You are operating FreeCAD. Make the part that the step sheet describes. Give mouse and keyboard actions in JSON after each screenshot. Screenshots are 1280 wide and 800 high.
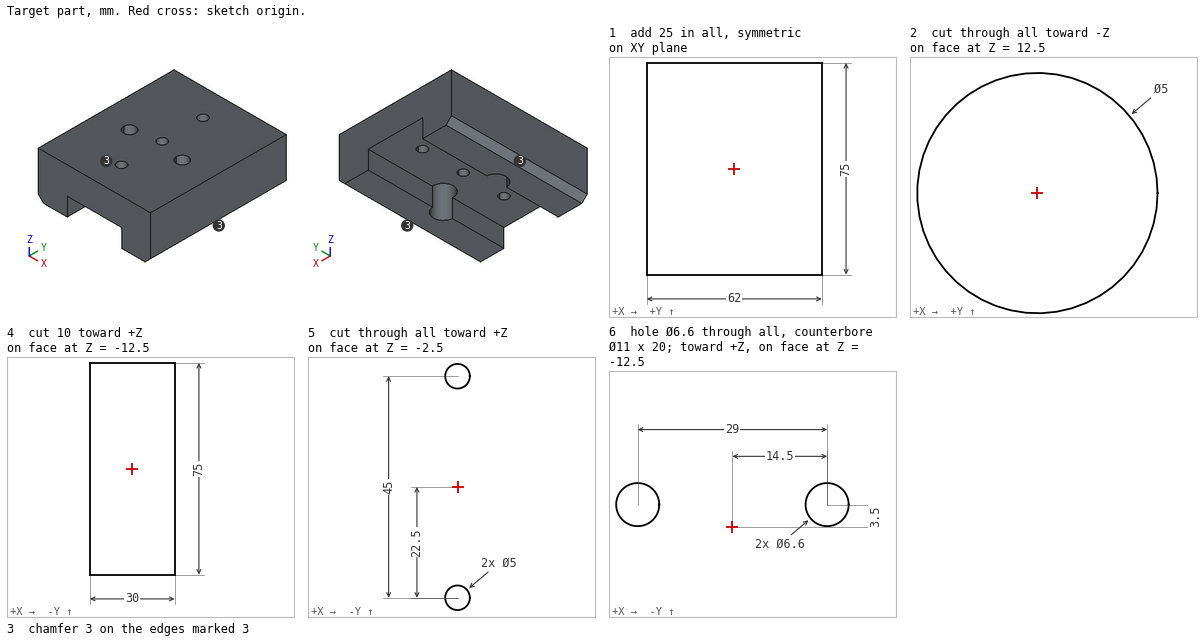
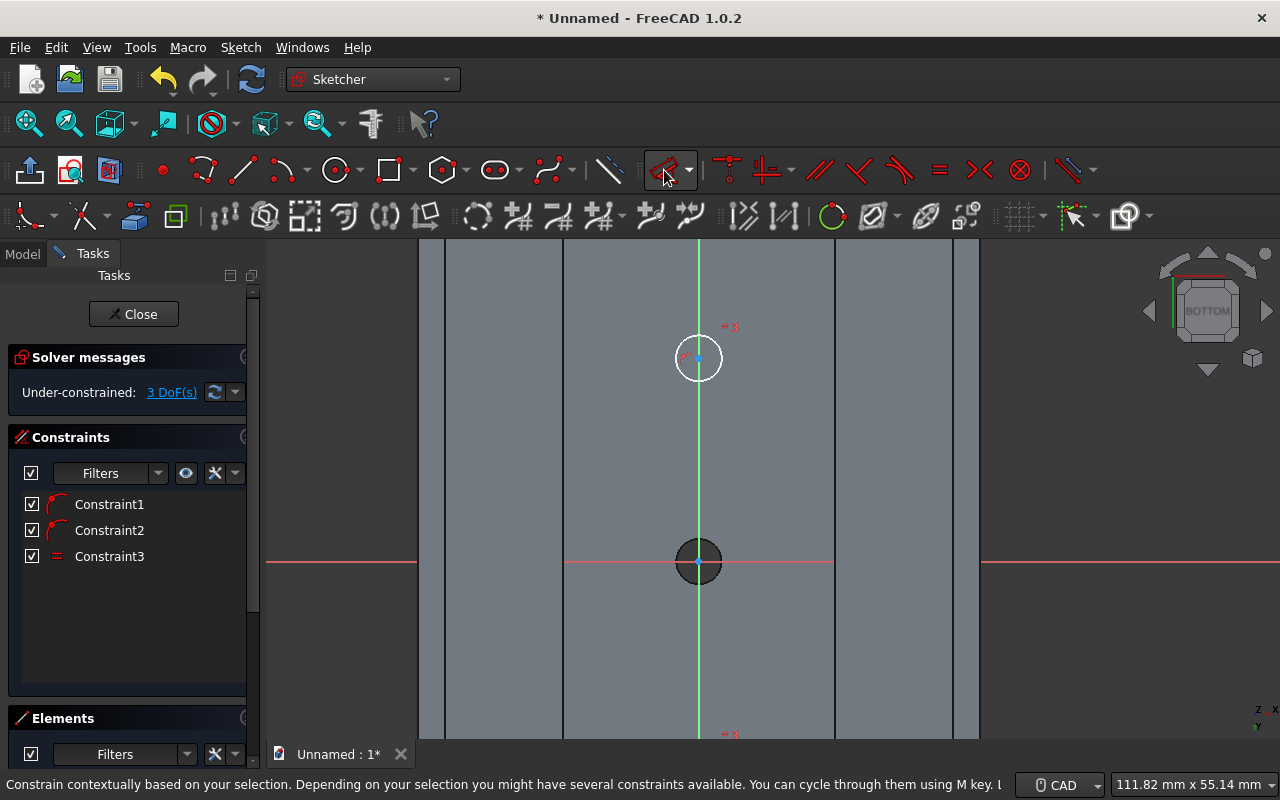
{"action": "scroll", "coordinate": [716, 341], "scroll_direction": "down", "scroll_amount": 2}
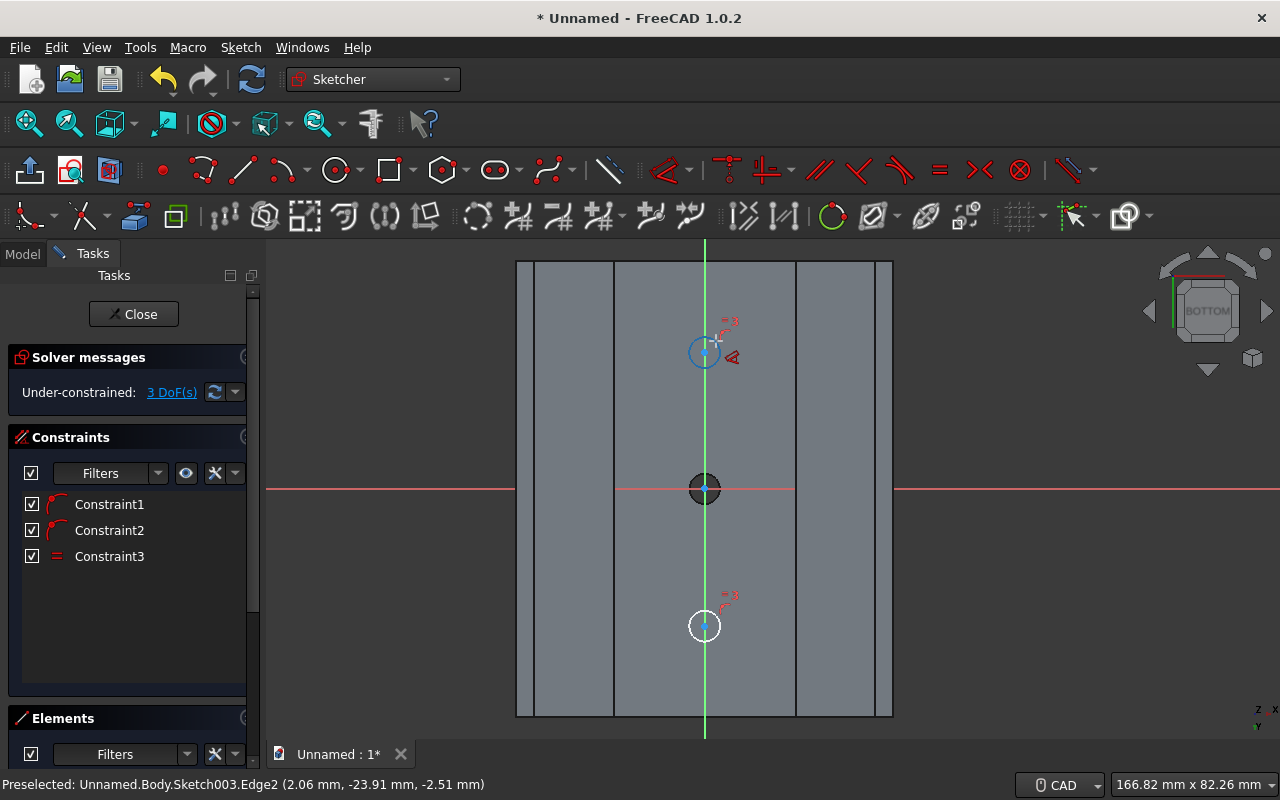
{"action": "scroll", "coordinate": [716, 615], "scroll_direction": "up", "scroll_amount": 2}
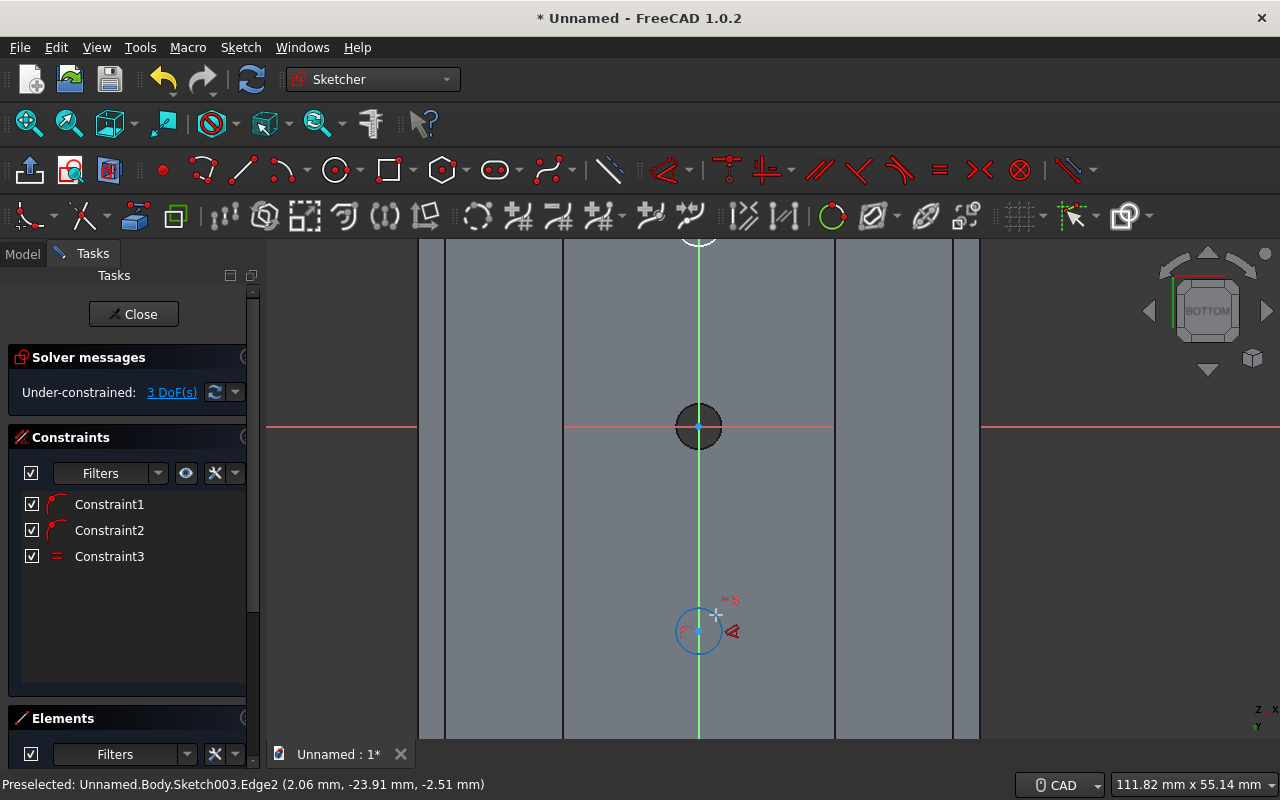
{"action": "left_click", "coordinate": [715, 615]}
{"action": "left_click", "coordinate": [737, 592]}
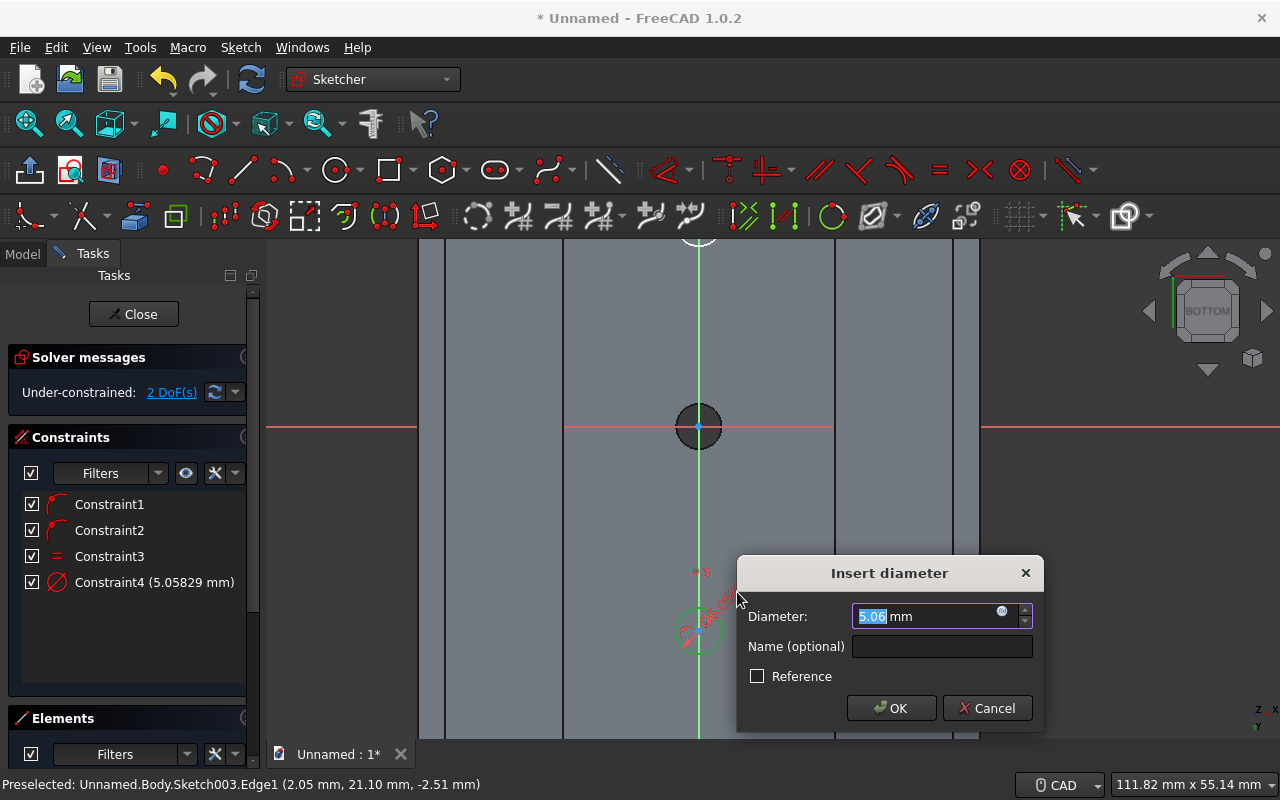
{"action": "type", "text": "5"}
{"action": "key", "text": "Return"}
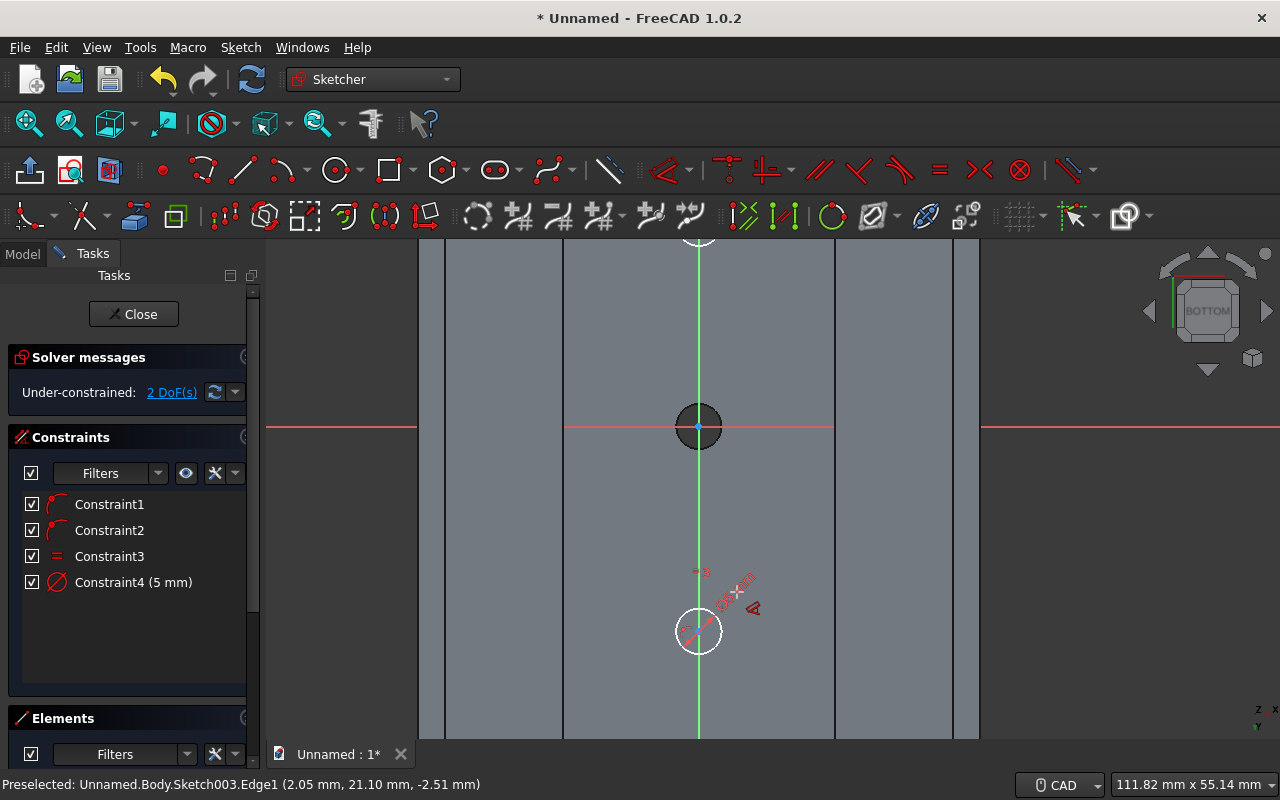
{"action": "left_click", "coordinate": [699, 631]}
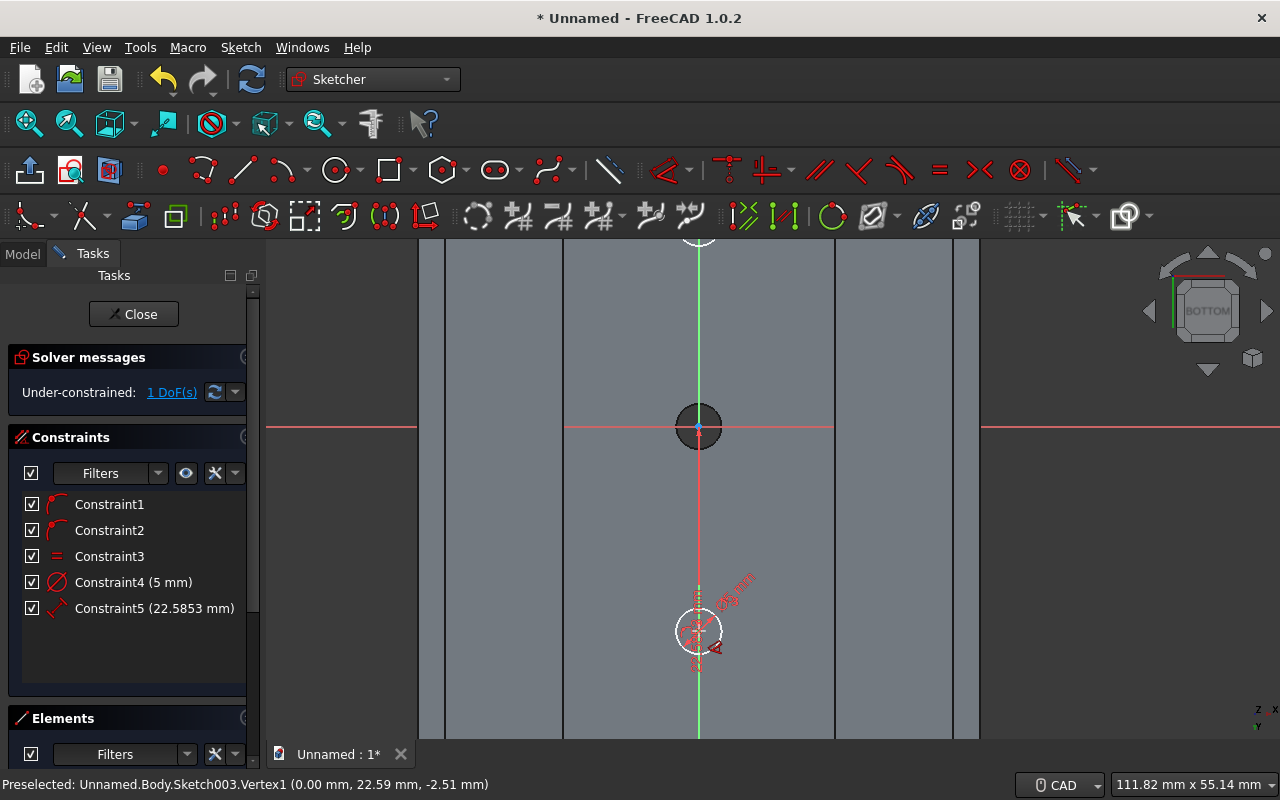
{"action": "scroll", "coordinate": [716, 616], "scroll_direction": "down", "scroll_amount": 2}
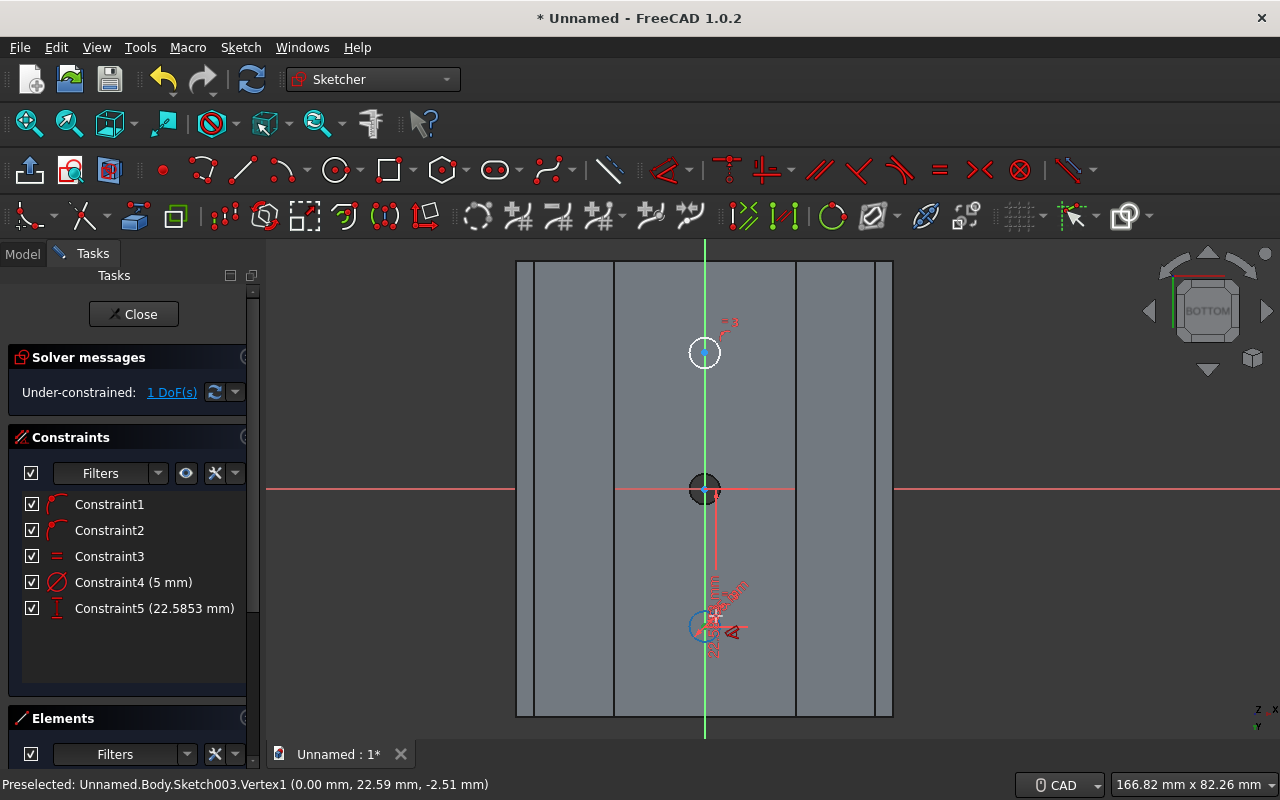
{"action": "left_click", "coordinate": [705, 353]}
{"action": "left_click", "coordinate": [739, 427]}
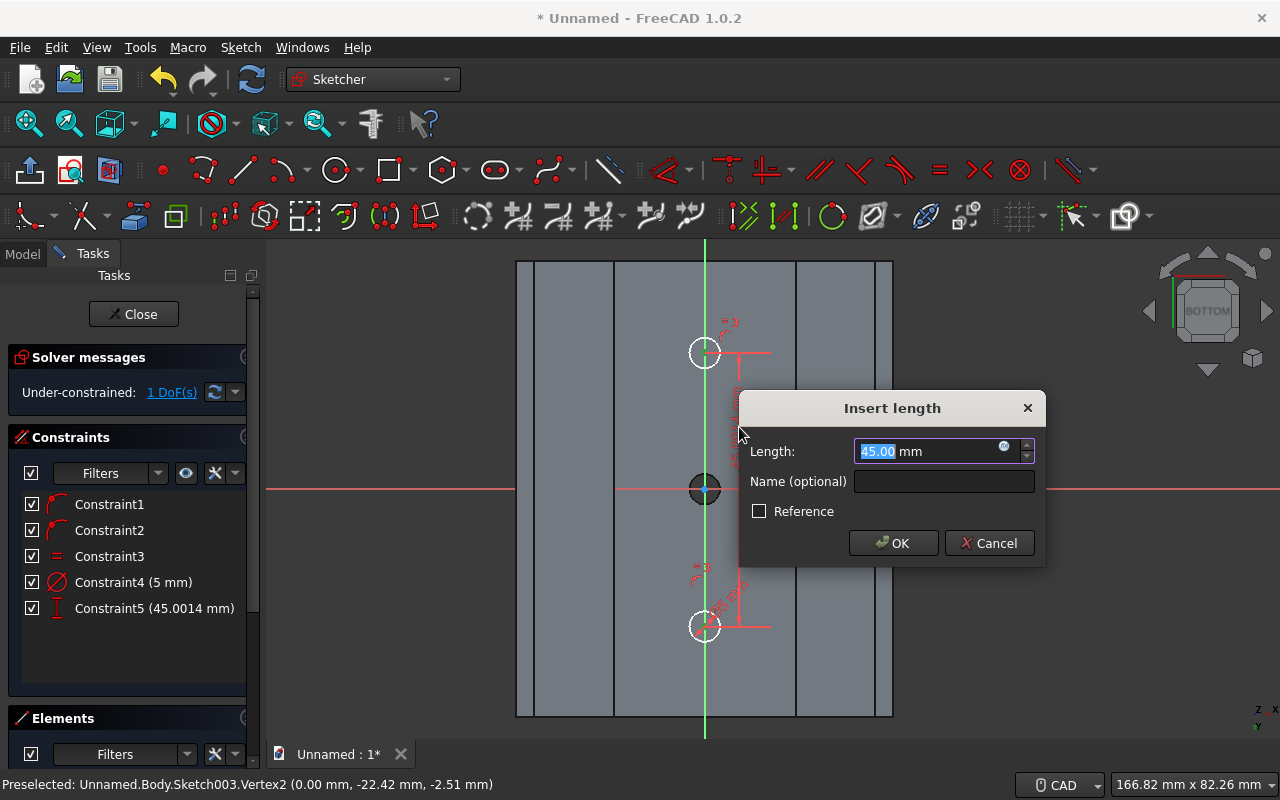
{"action": "type", "text": "45"}
{"action": "key", "text": "Return"}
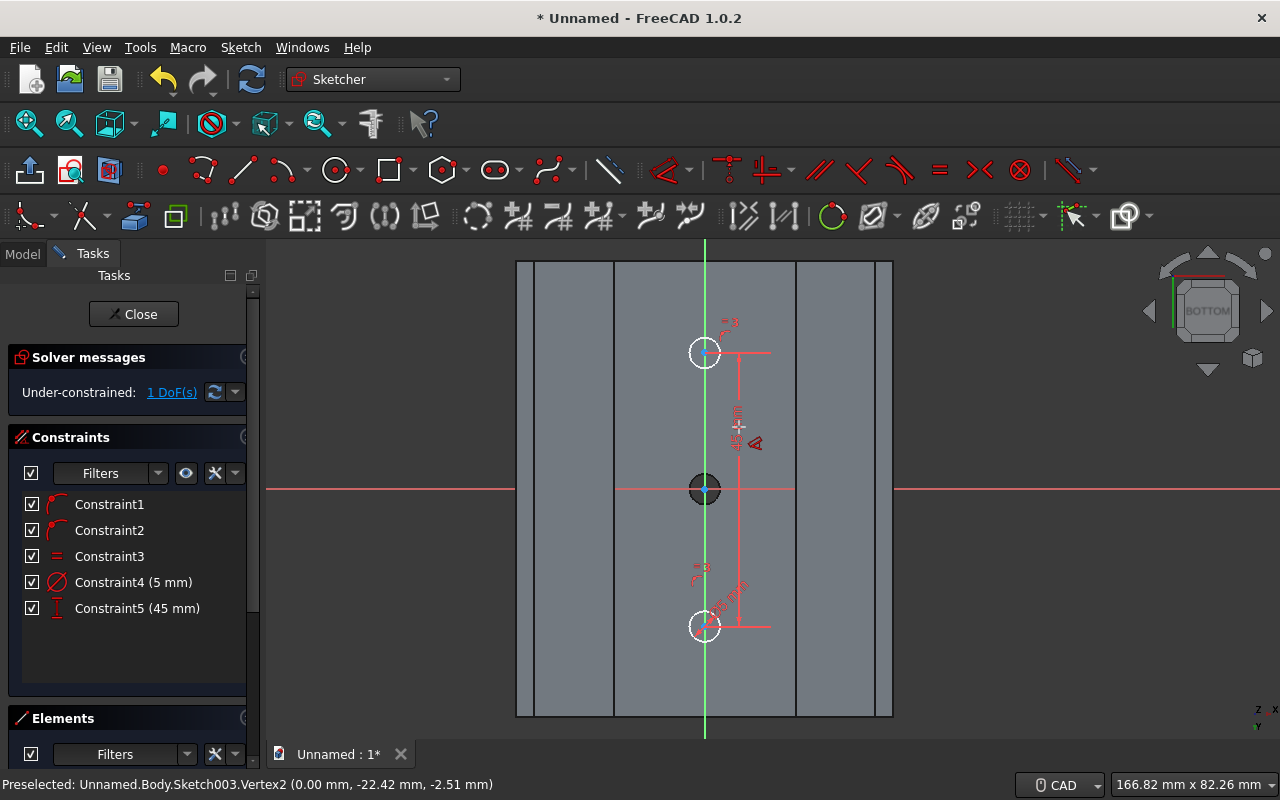
{"action": "left_click", "coordinate": [705, 627]}
{"action": "left_click", "coordinate": [739, 558]}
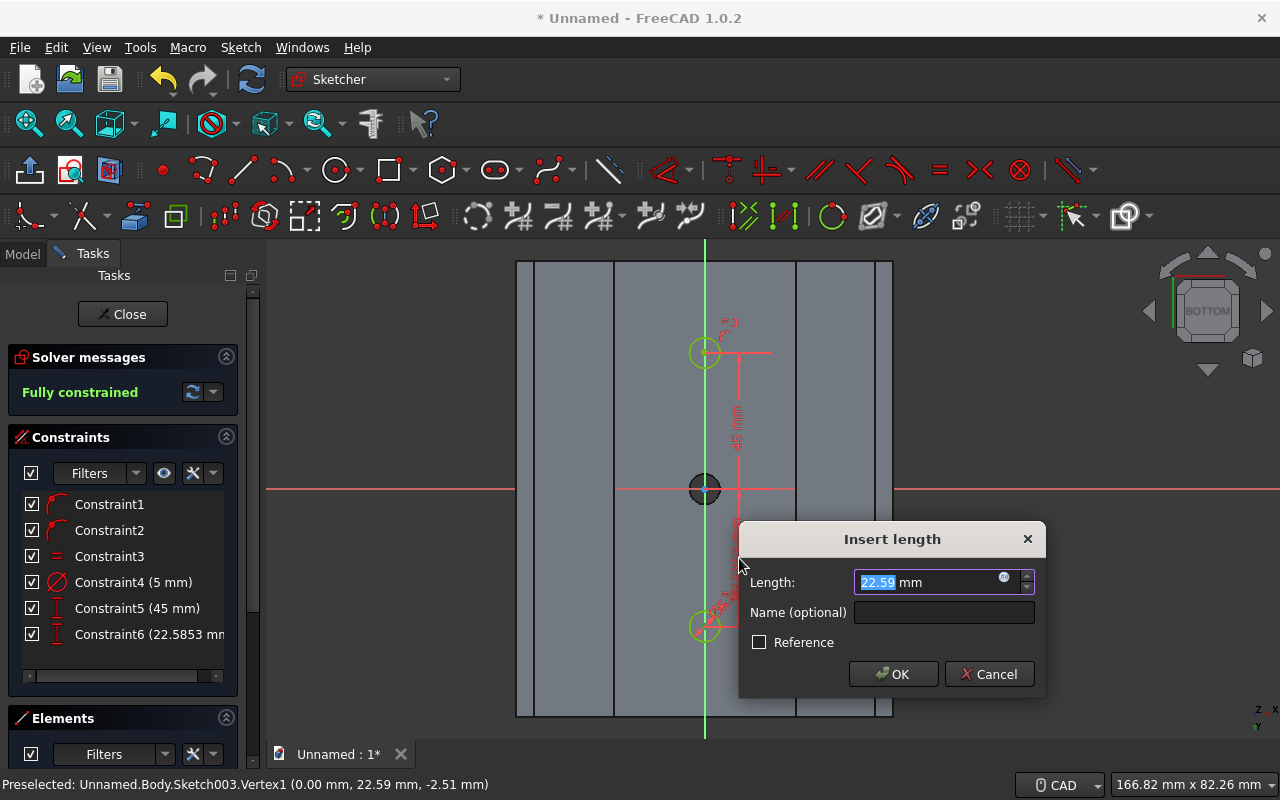
{"action": "type", "text": "22.5"}
{"action": "key", "text": "Return"}
{"action": "key", "text": "Escape"}